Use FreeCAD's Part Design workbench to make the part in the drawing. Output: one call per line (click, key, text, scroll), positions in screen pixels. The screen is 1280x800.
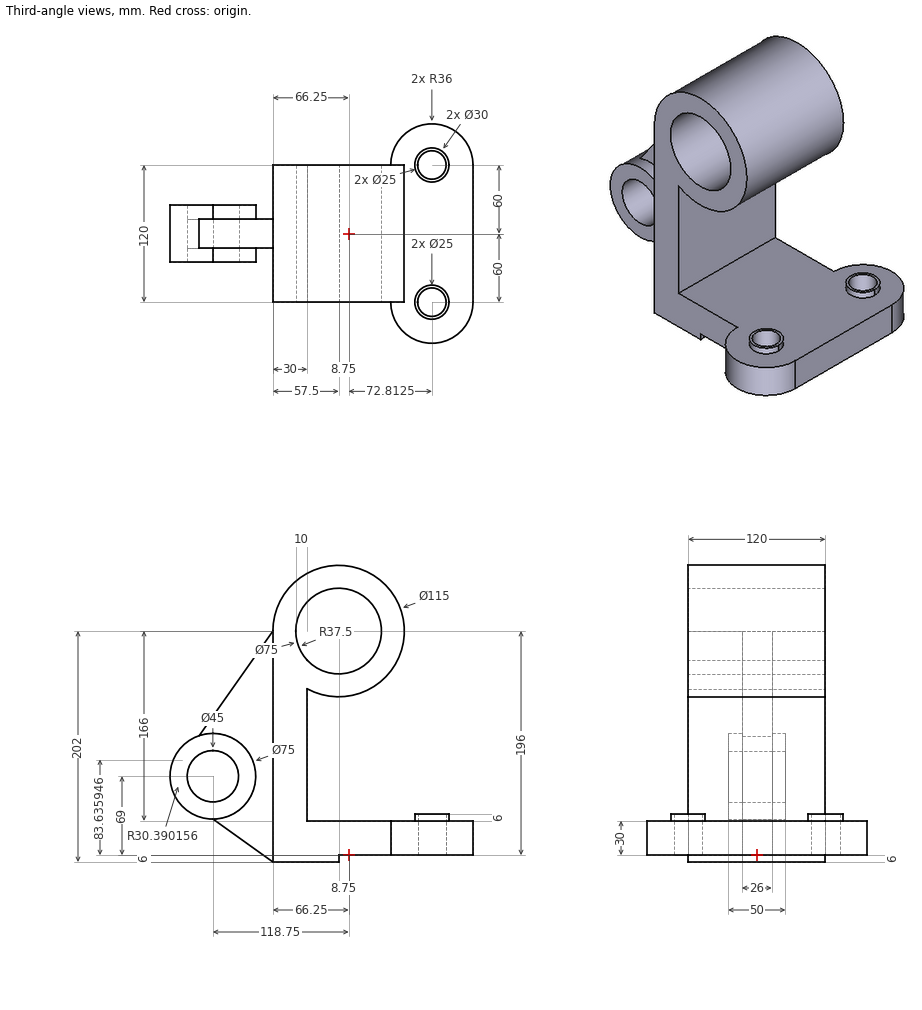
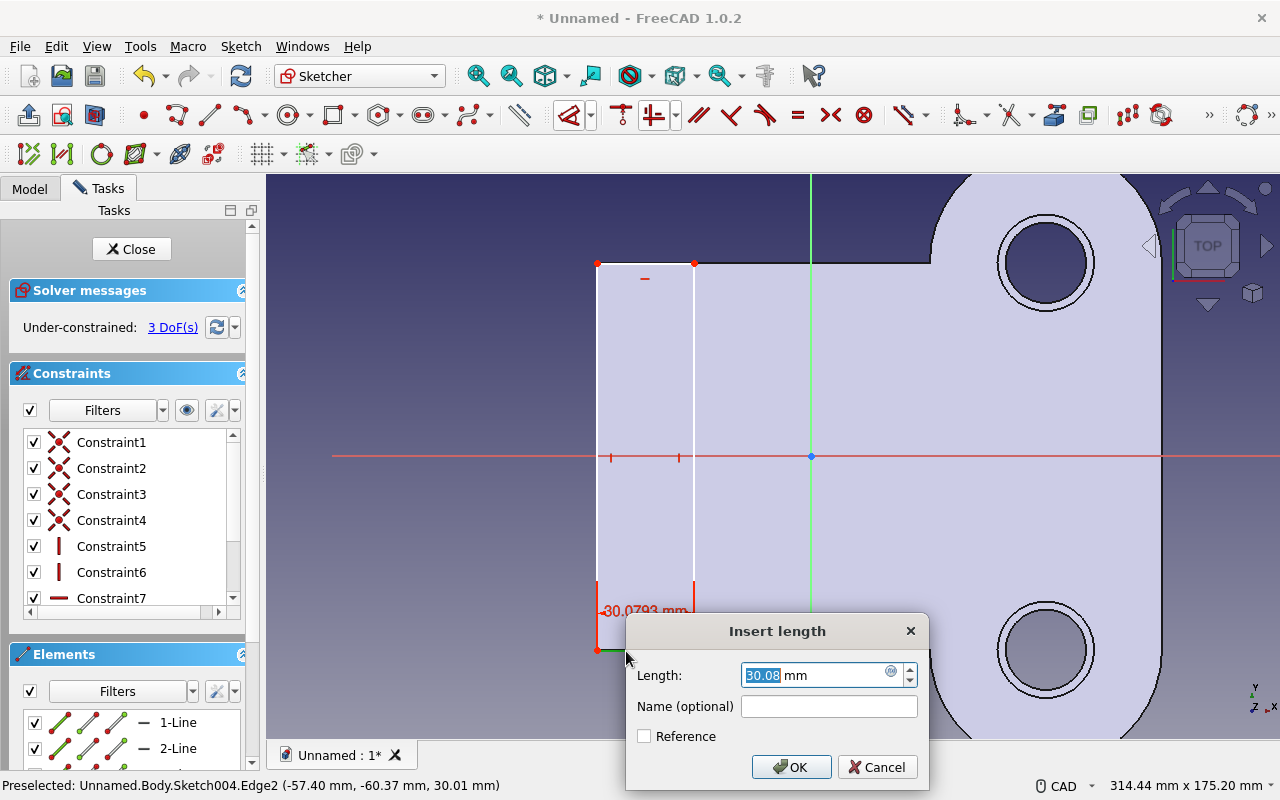
text(30)
key(Return)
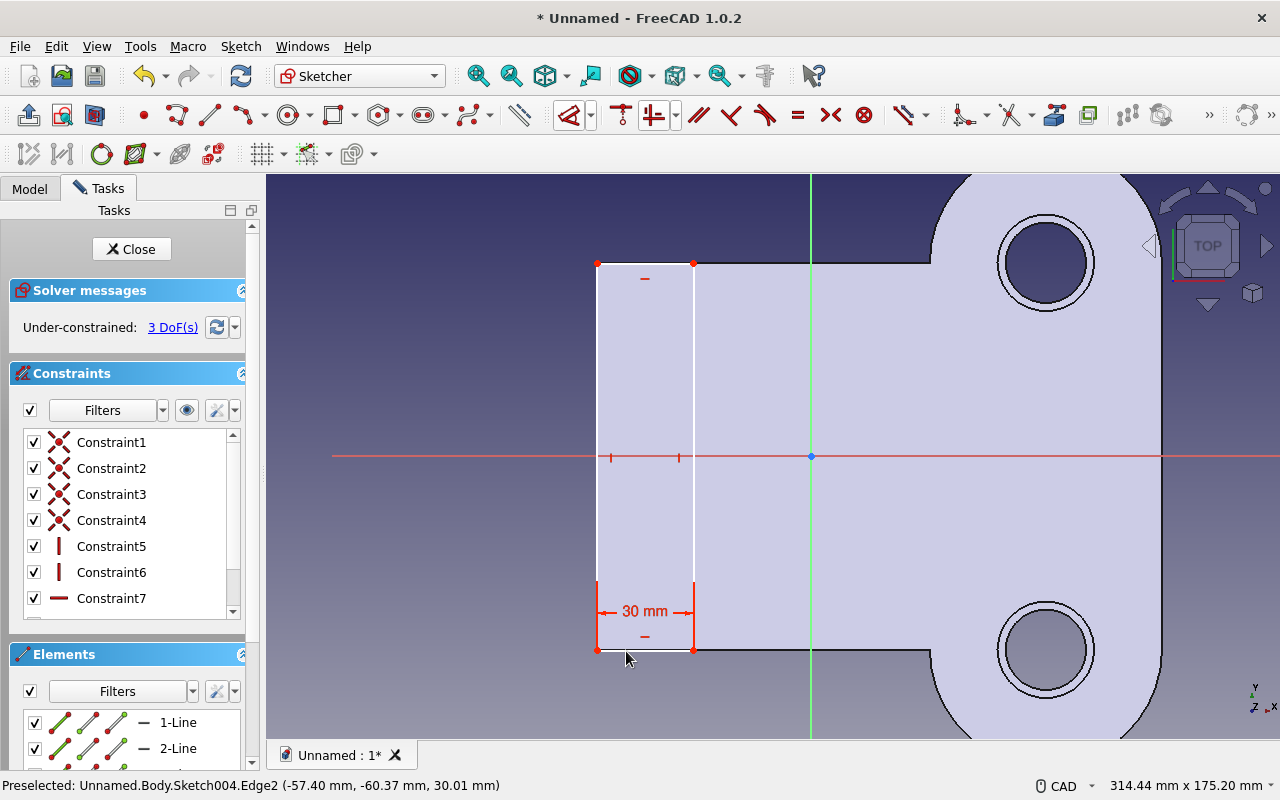
click(597, 380)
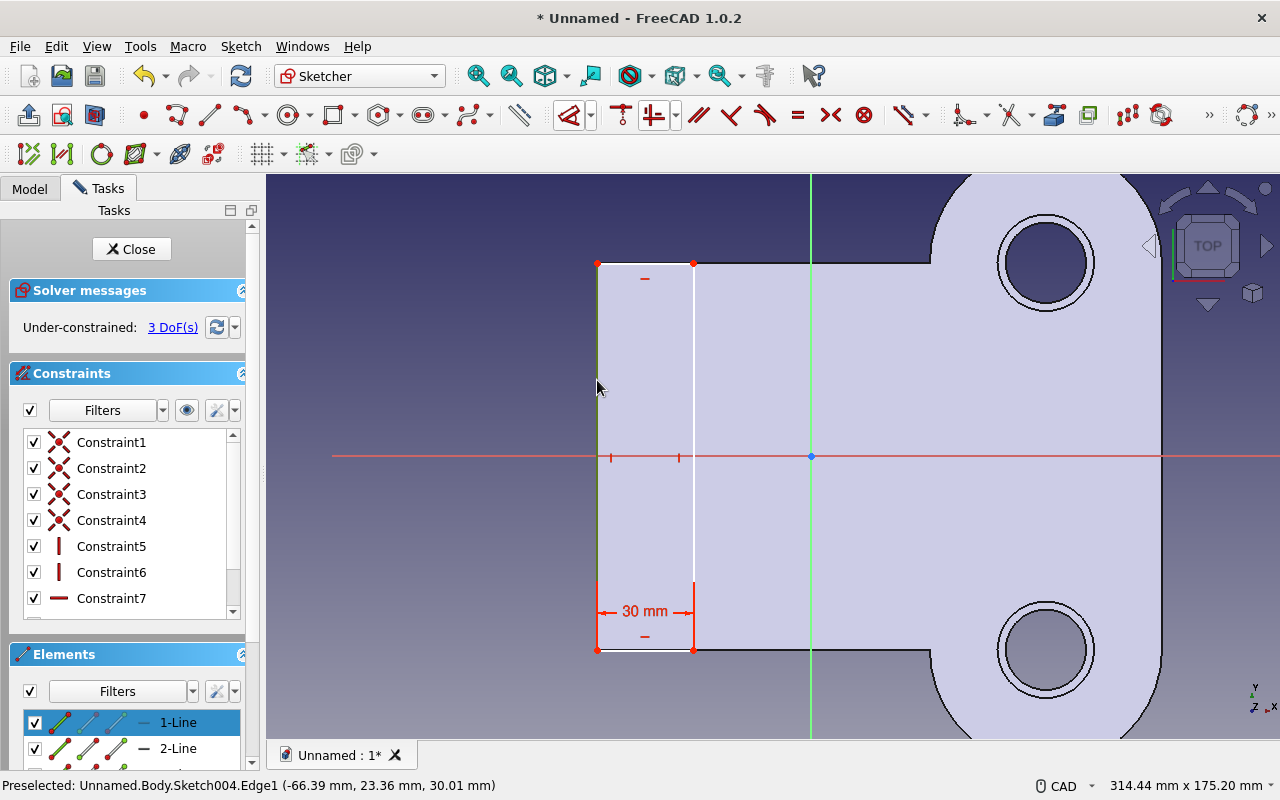
key(i)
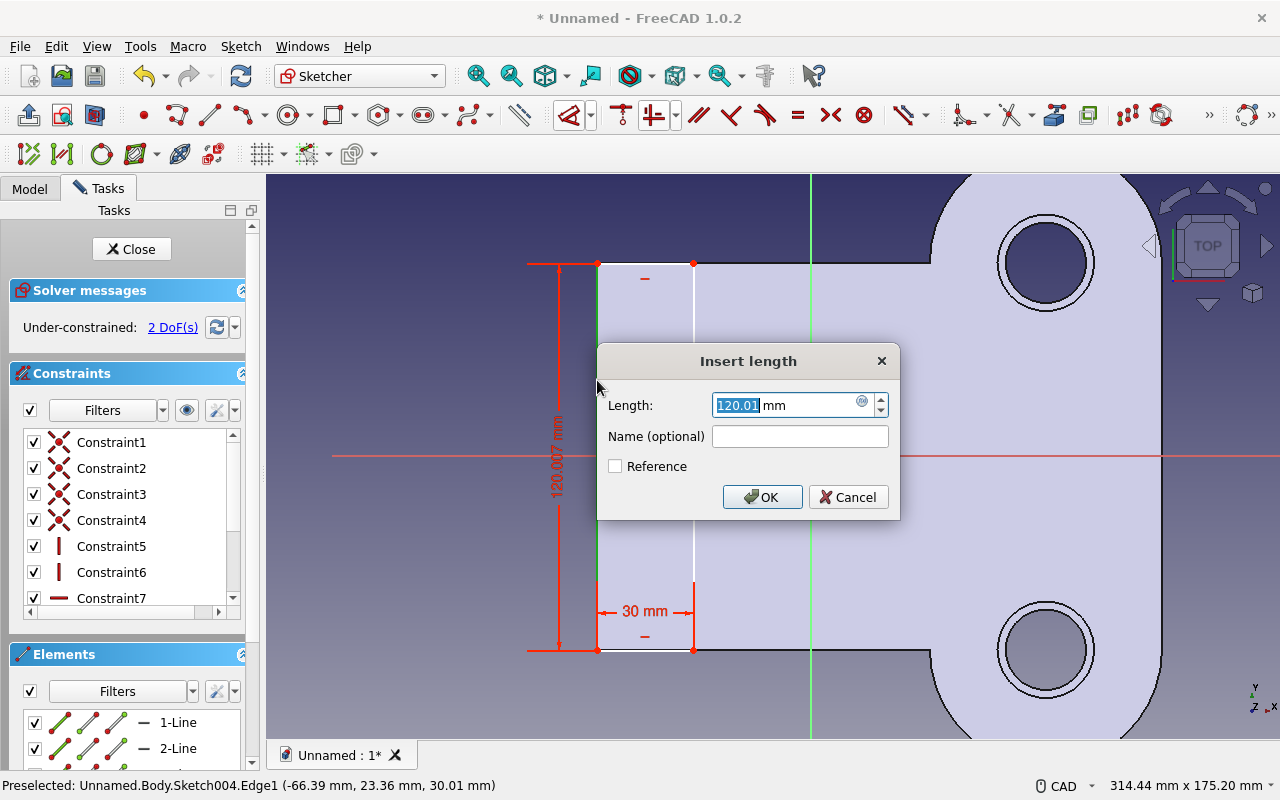
text(120)
key(Return)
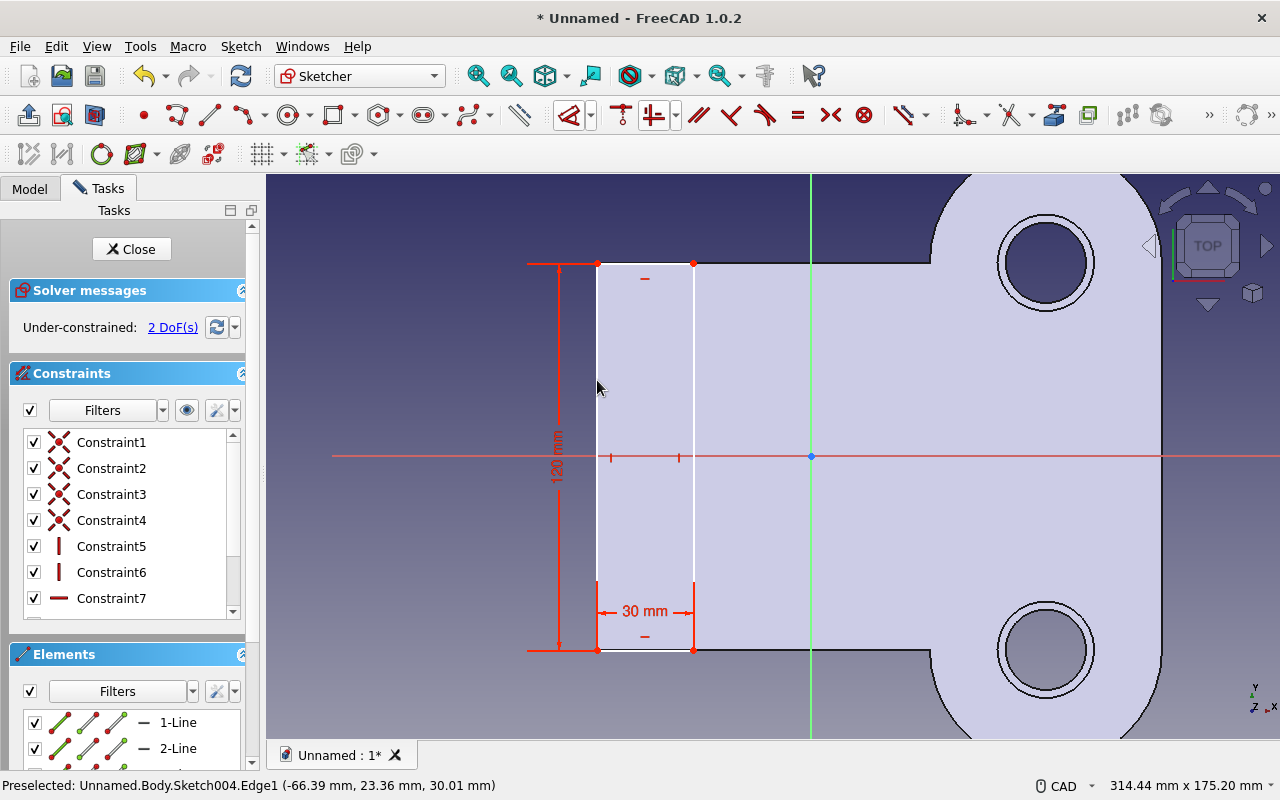
click(597, 264)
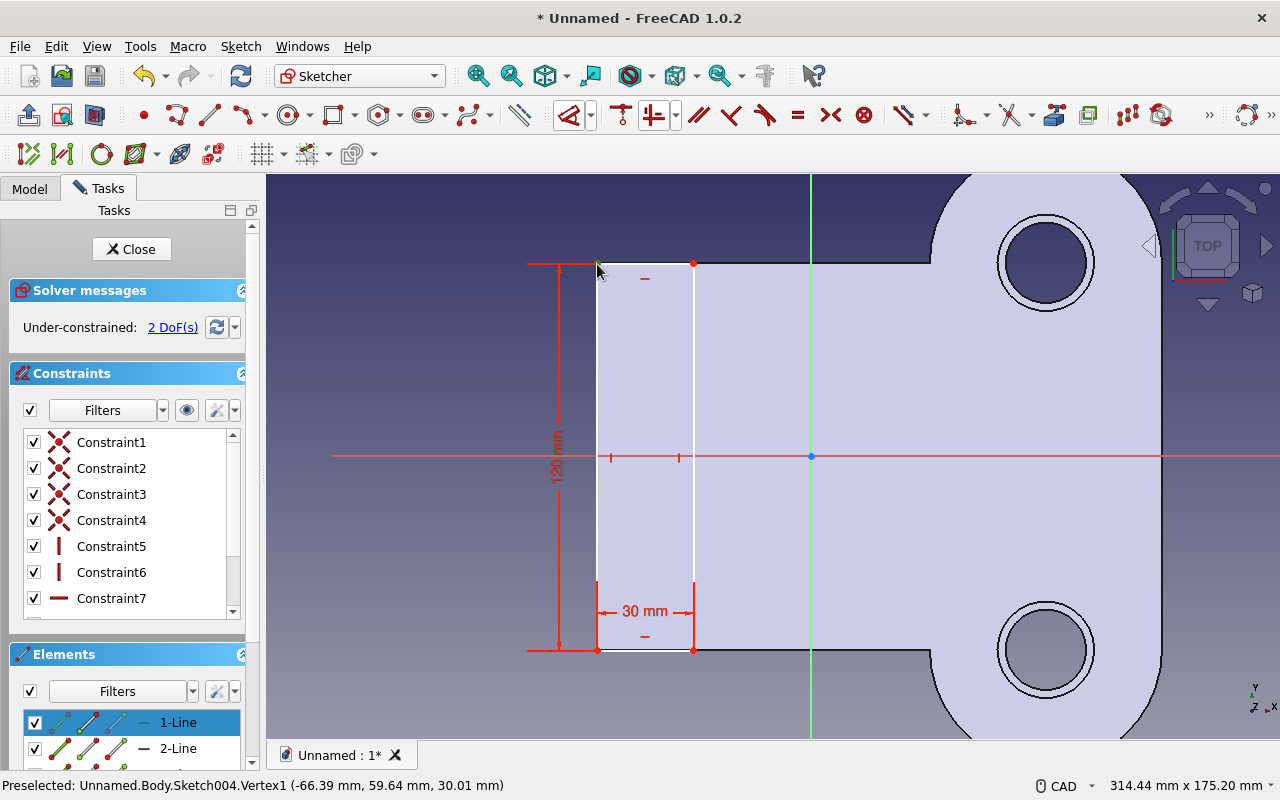
key(i)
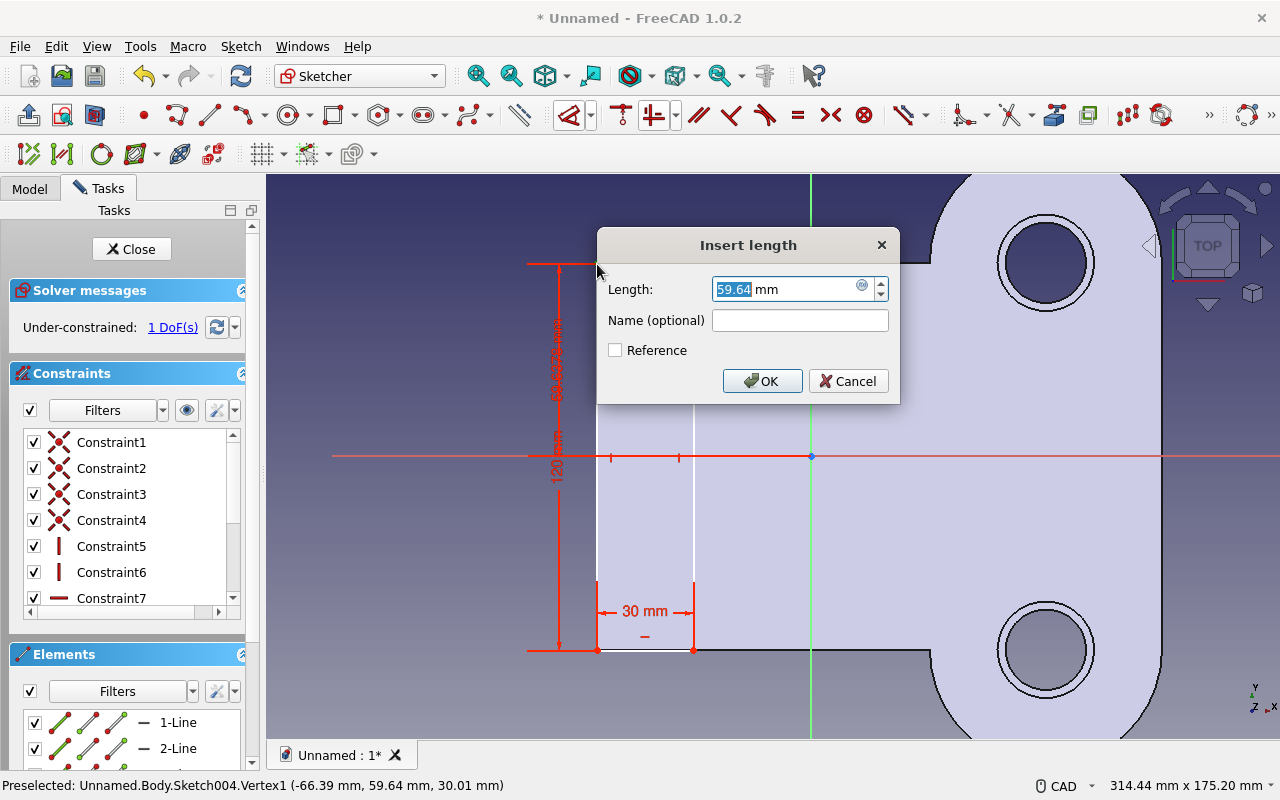
text(60)
key(Return)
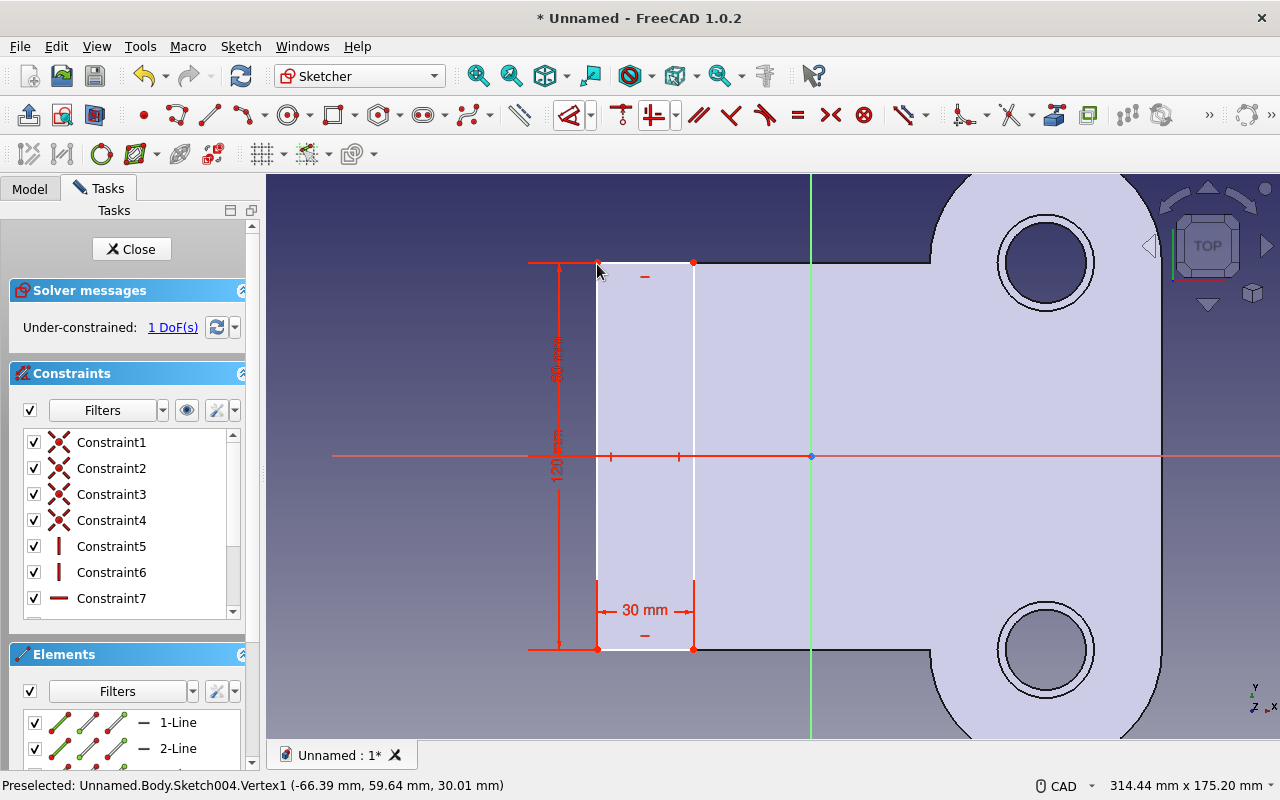
click(597, 263)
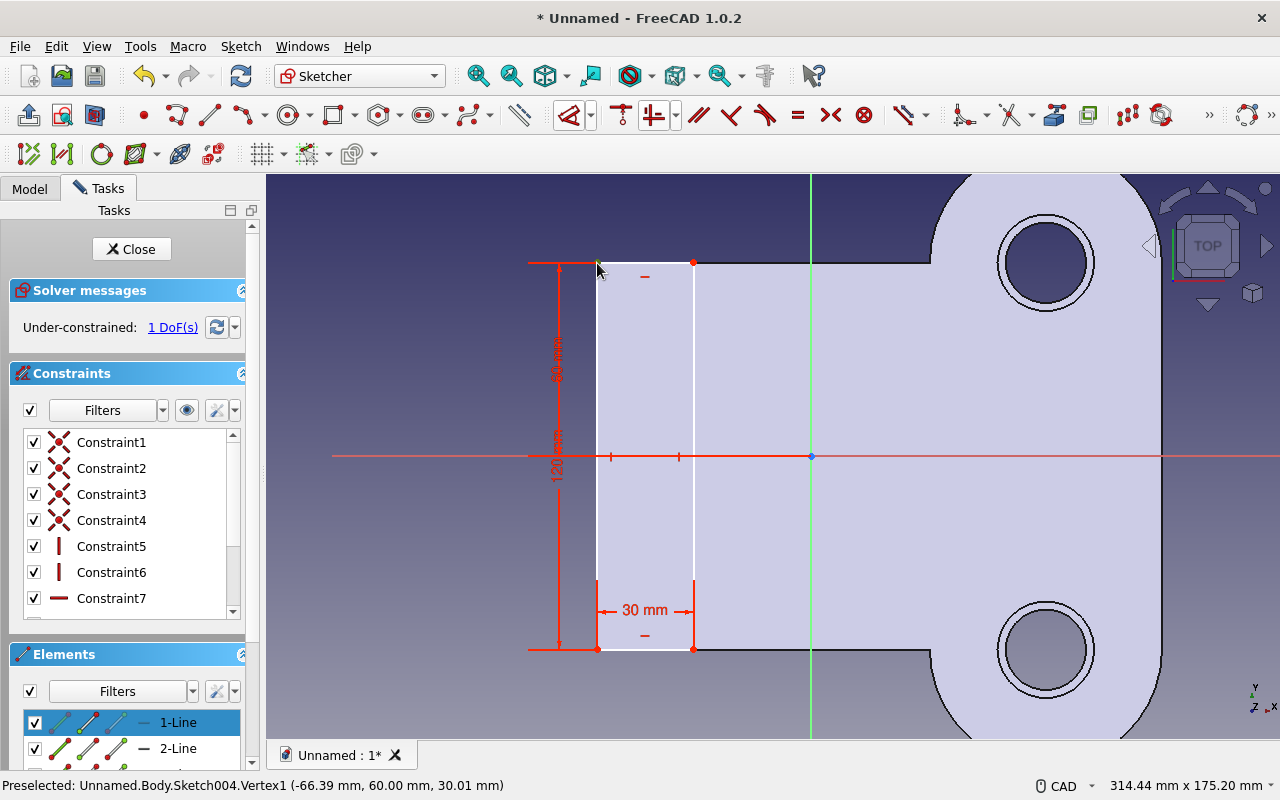
key(l)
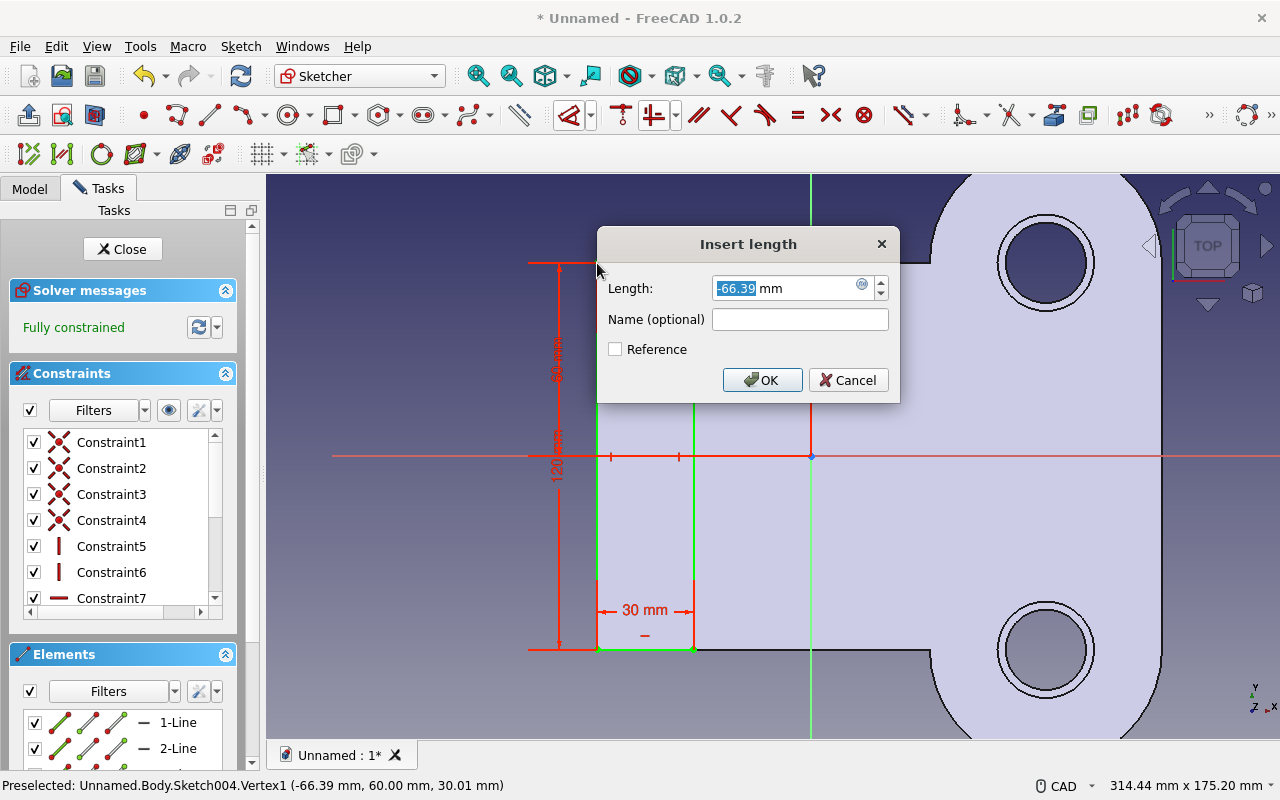
text(-66.25)
key(Return)